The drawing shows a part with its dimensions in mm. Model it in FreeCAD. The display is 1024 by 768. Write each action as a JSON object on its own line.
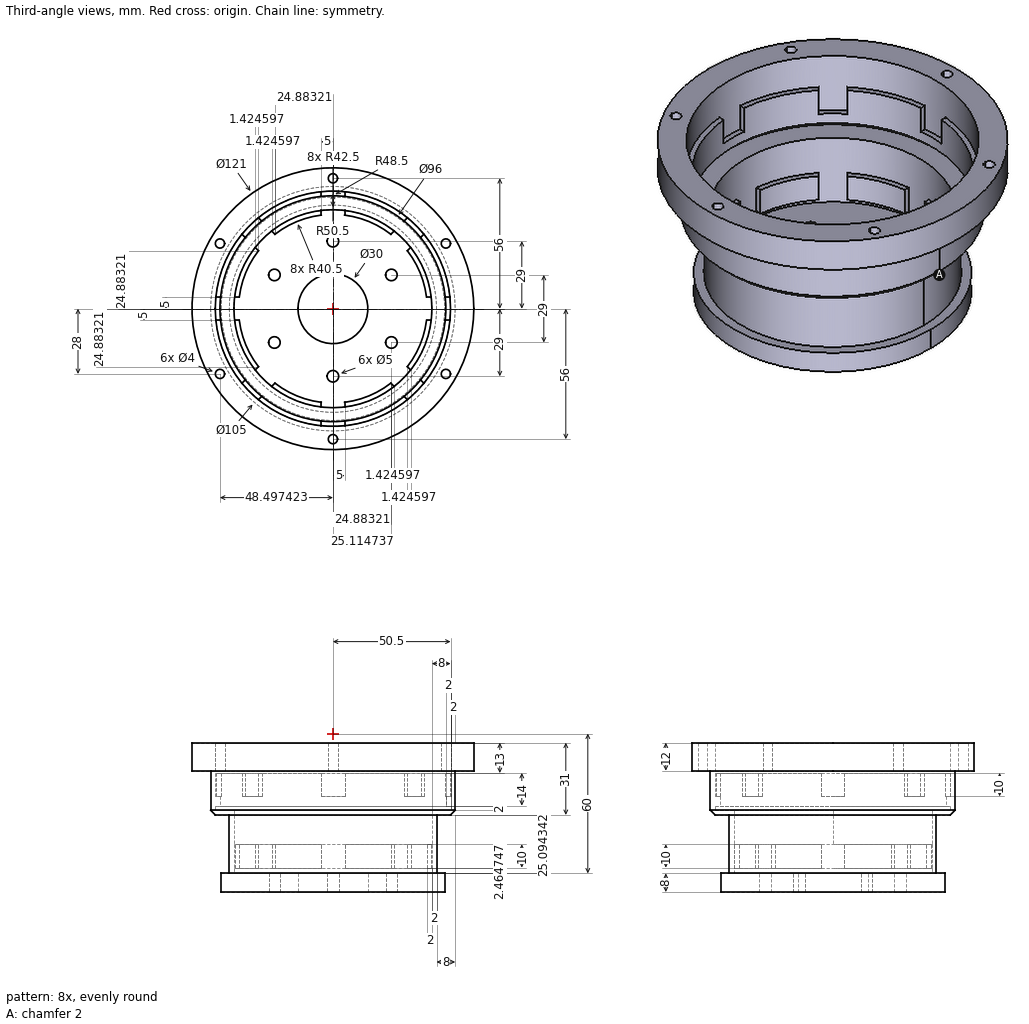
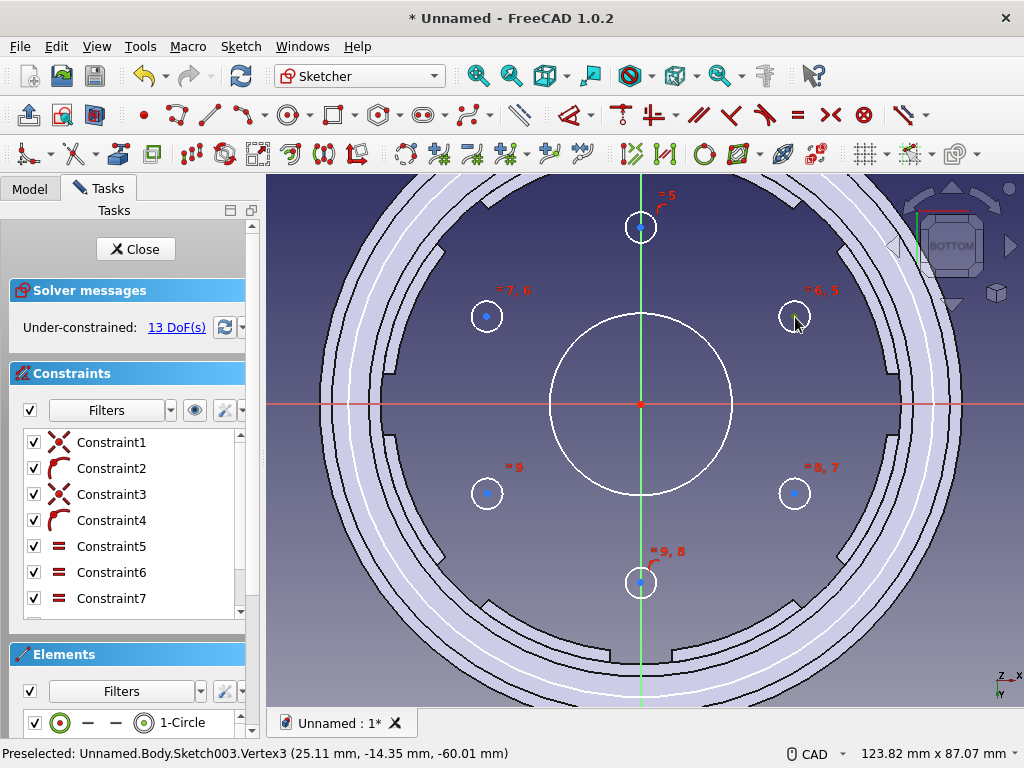
{"action": "left_click", "coordinate": [487, 317]}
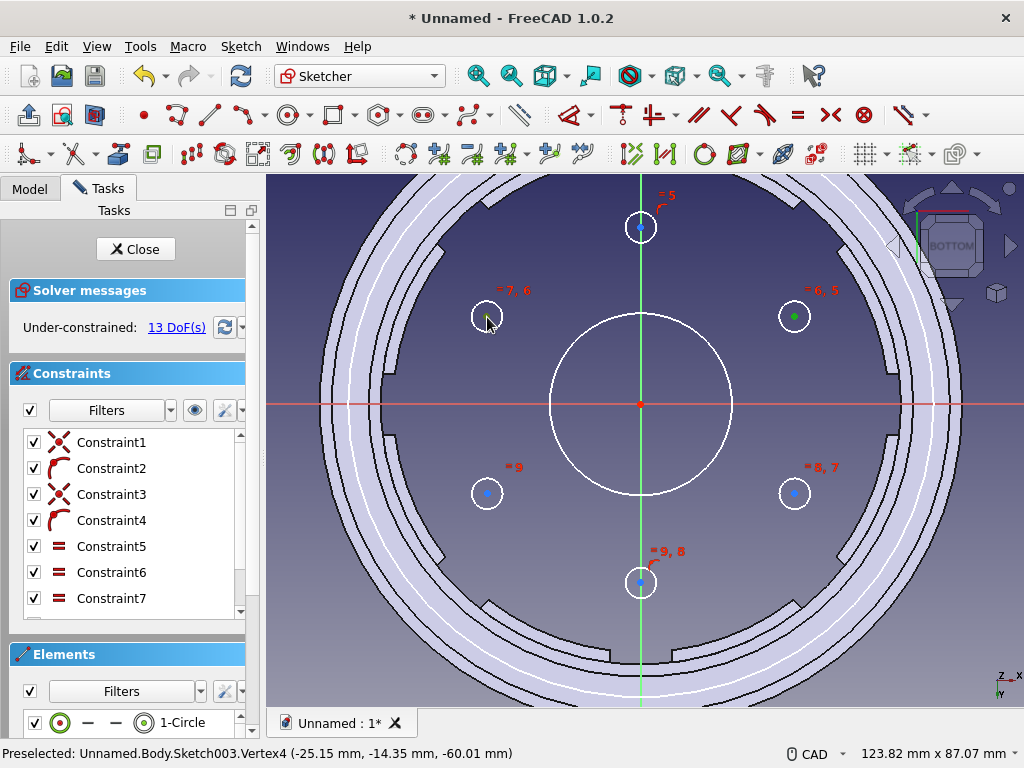
{"action": "left_click", "coordinate": [641, 645]}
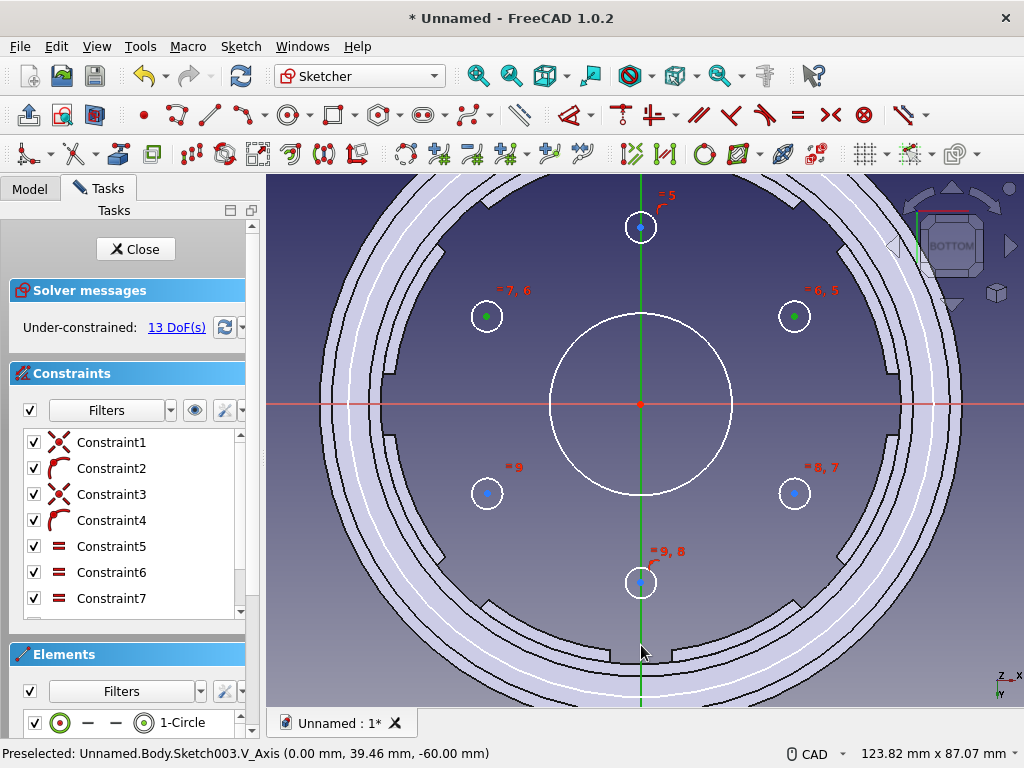
{"action": "left_click", "coordinate": [831, 116]}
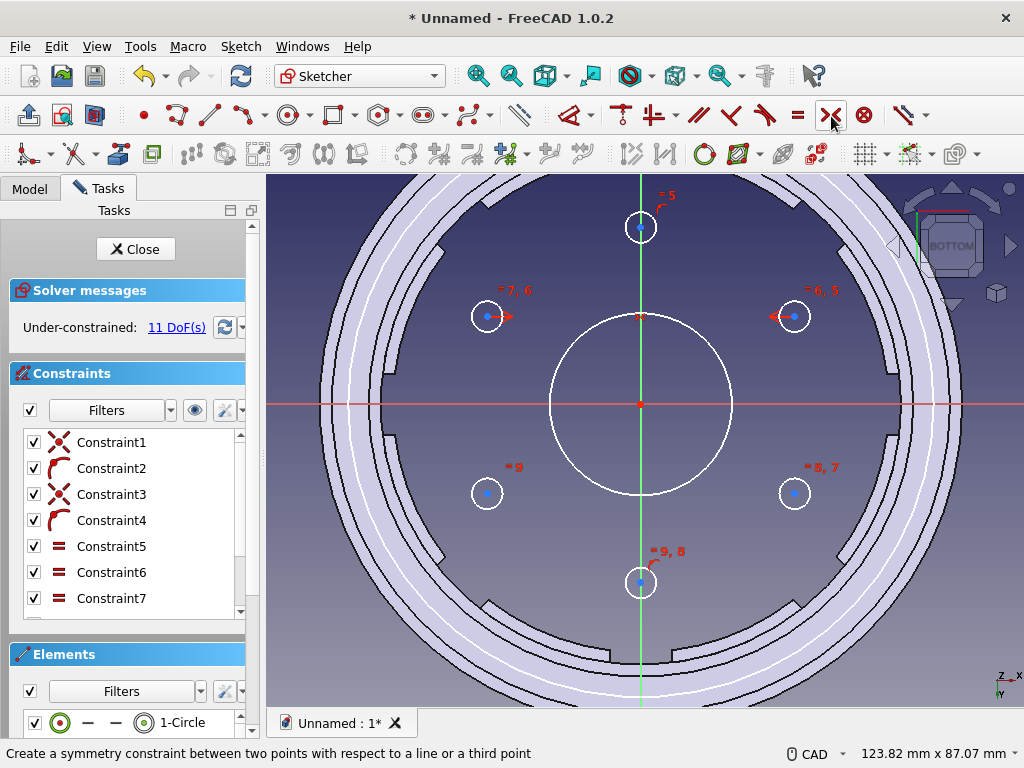
{"action": "left_click", "coordinate": [795, 317]}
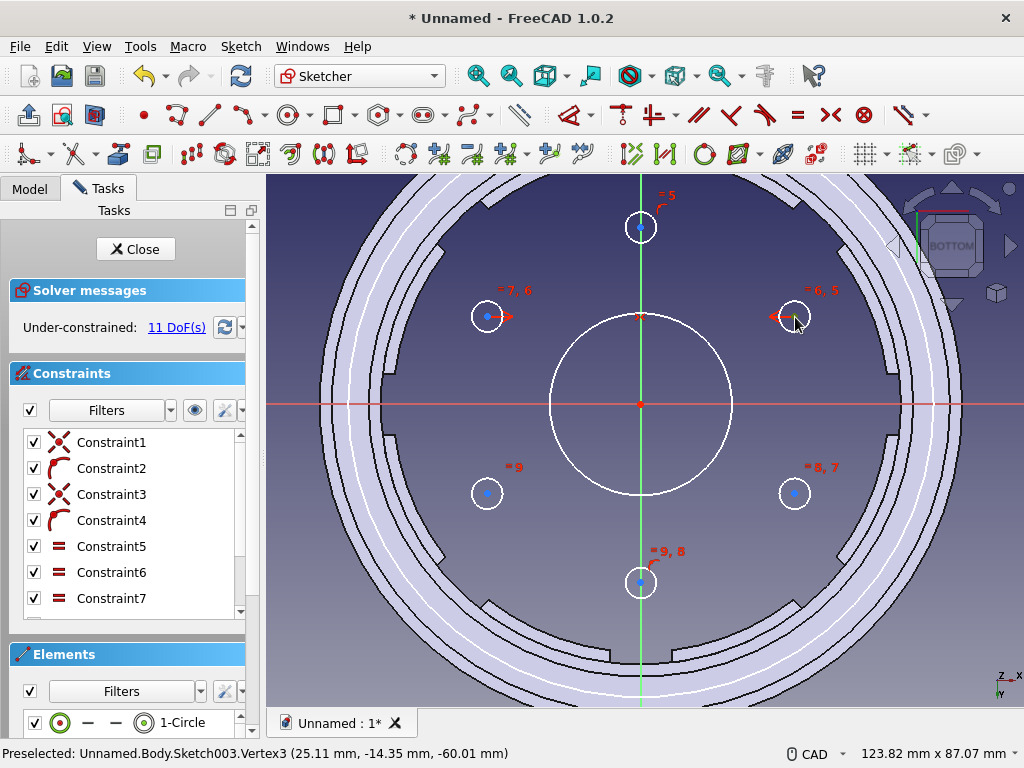
{"action": "left_click", "coordinate": [795, 494]}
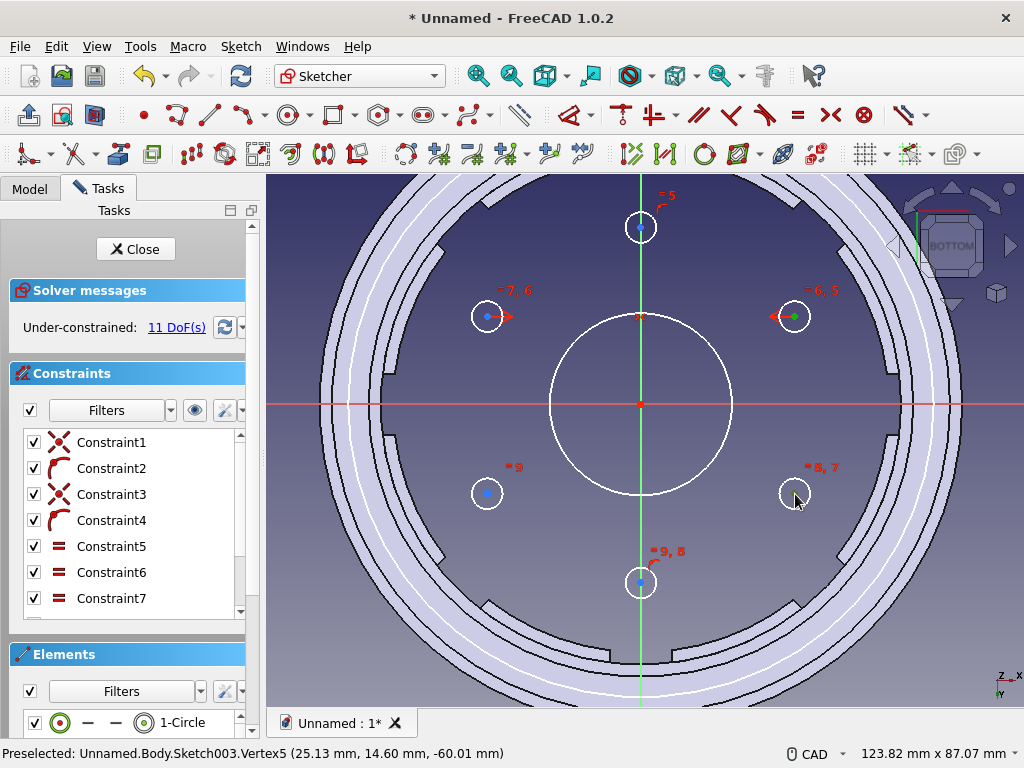
{"action": "left_click", "coordinate": [415, 404]}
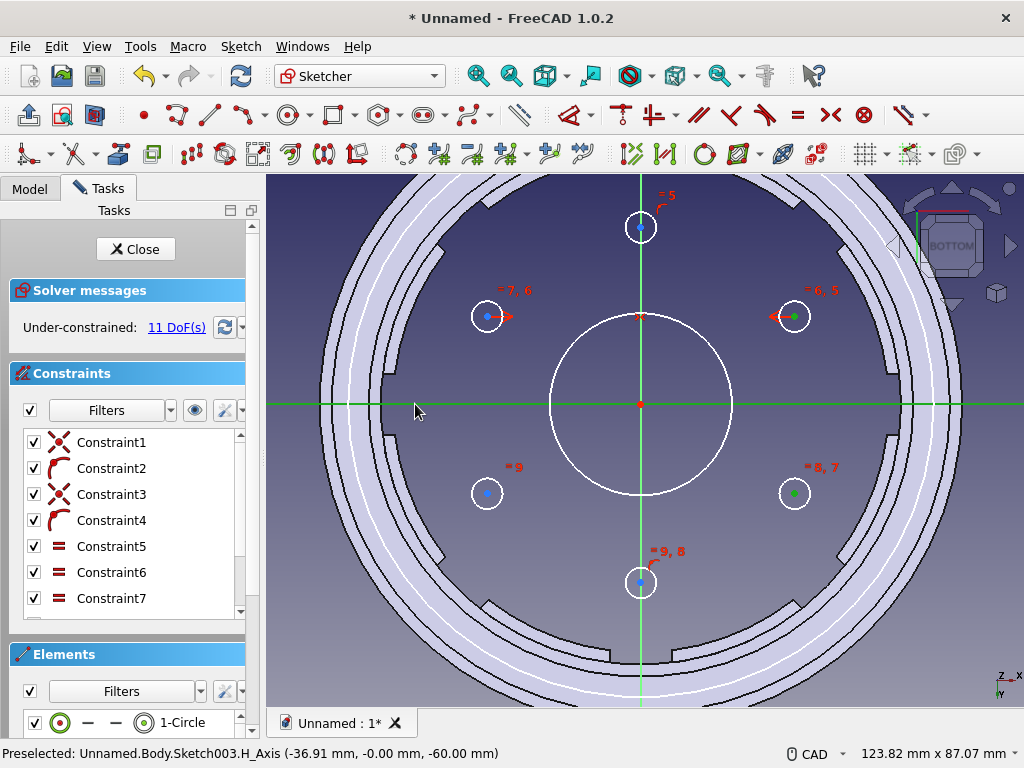
{"action": "left_click", "coordinate": [831, 116]}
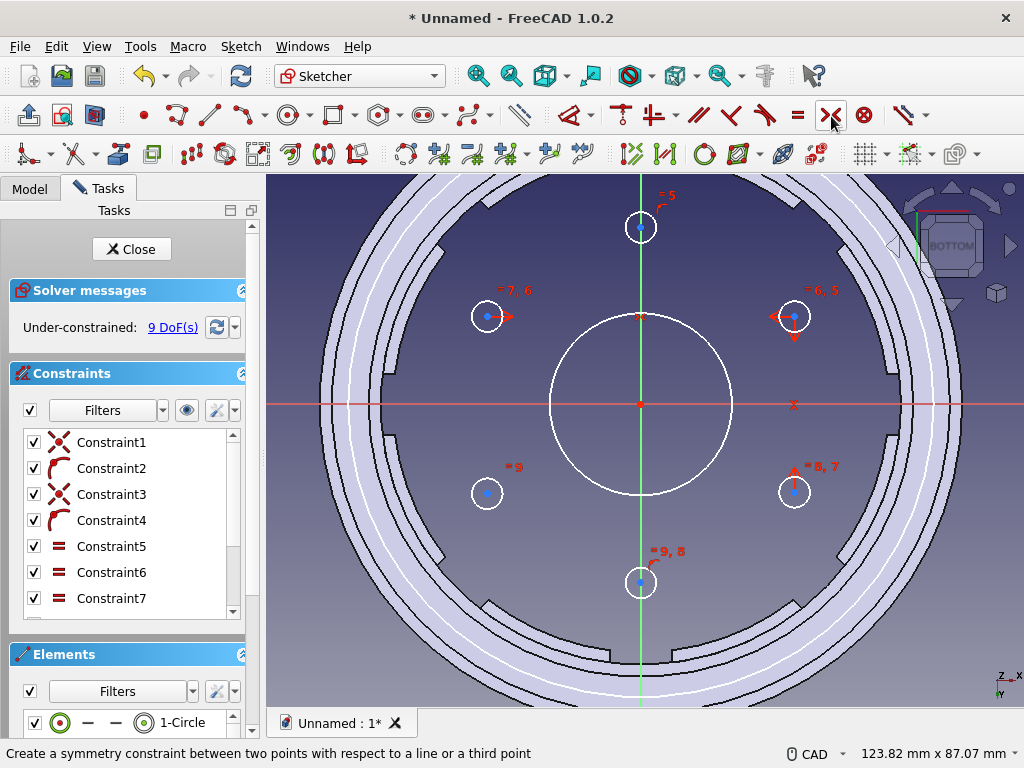
{"action": "left_click", "coordinate": [487, 317]}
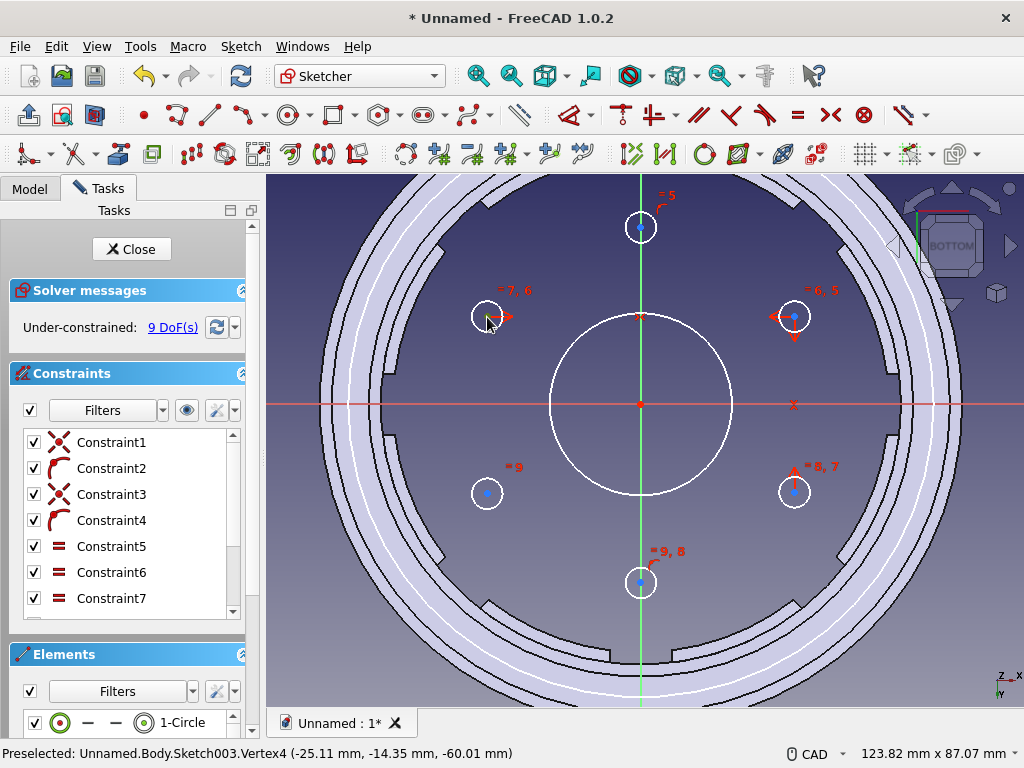
{"action": "left_click", "coordinate": [487, 494]}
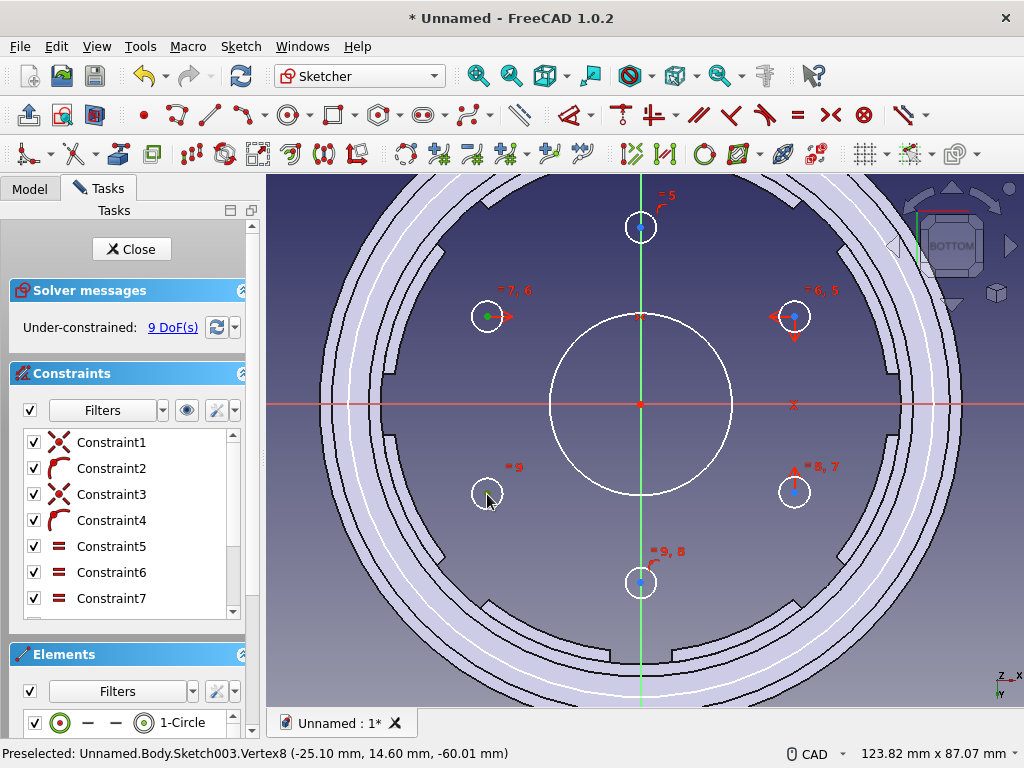
{"action": "left_click", "coordinate": [415, 404]}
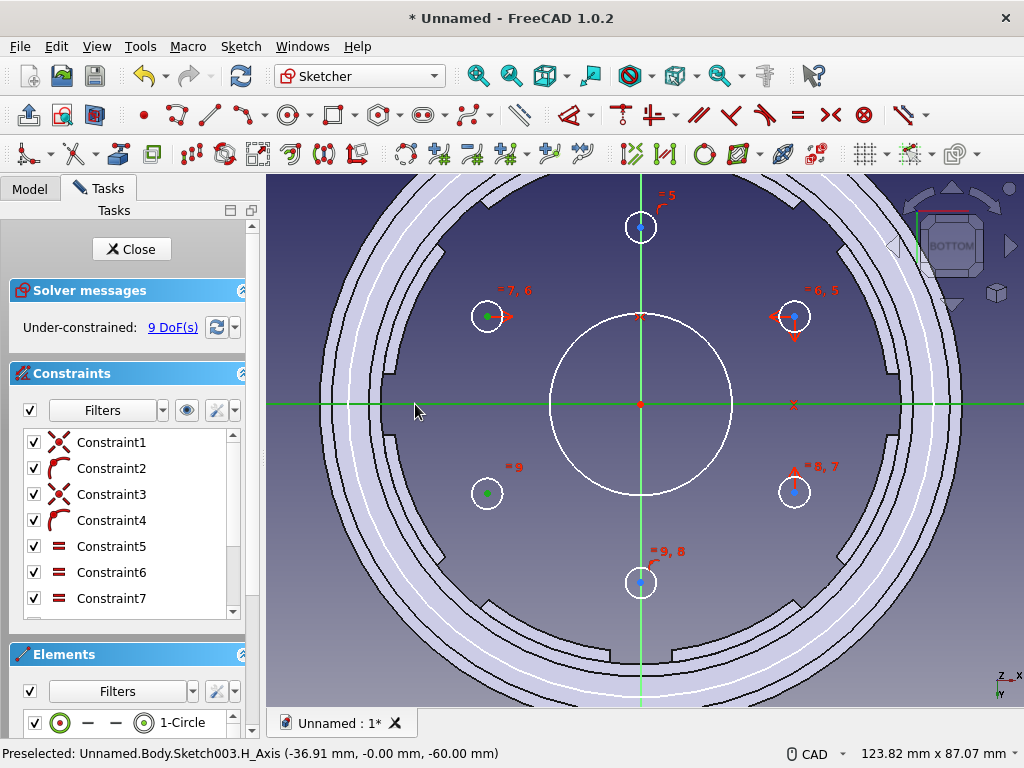
{"action": "left_click", "coordinate": [831, 116]}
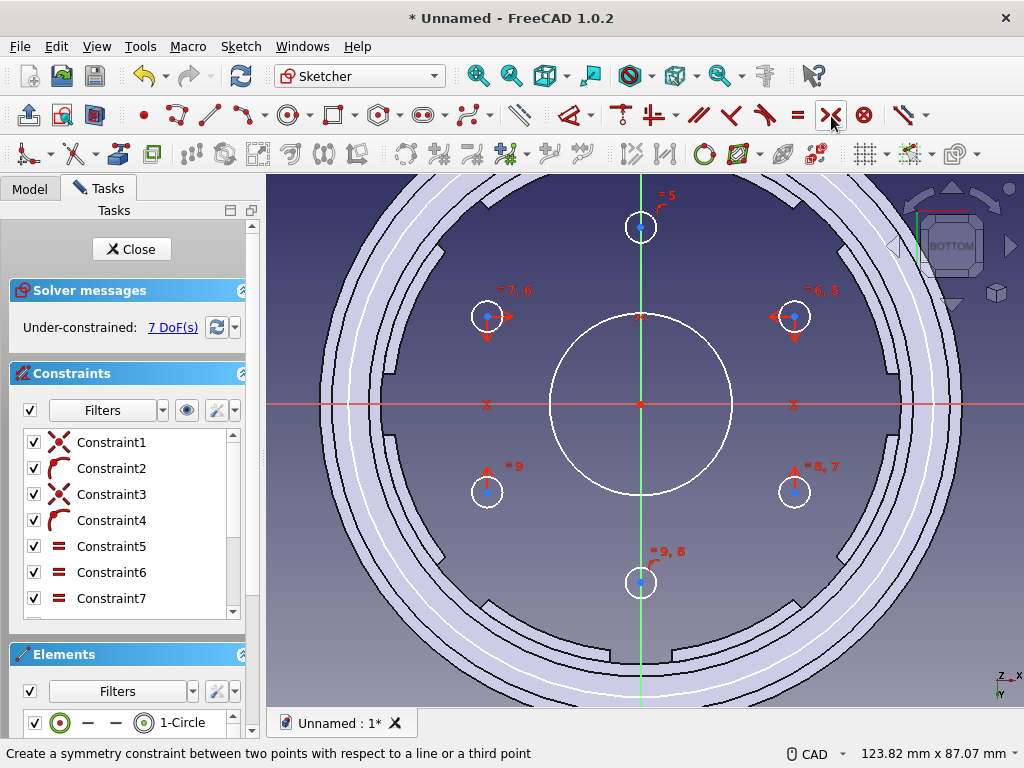
{"action": "left_click", "coordinate": [568, 116]}